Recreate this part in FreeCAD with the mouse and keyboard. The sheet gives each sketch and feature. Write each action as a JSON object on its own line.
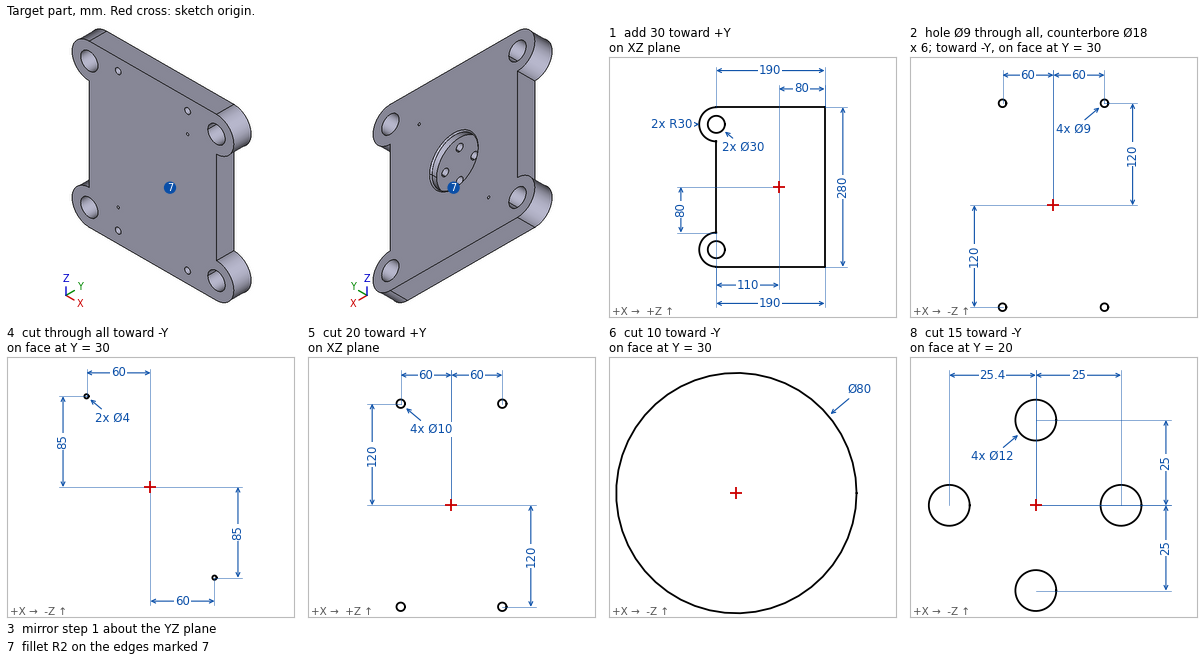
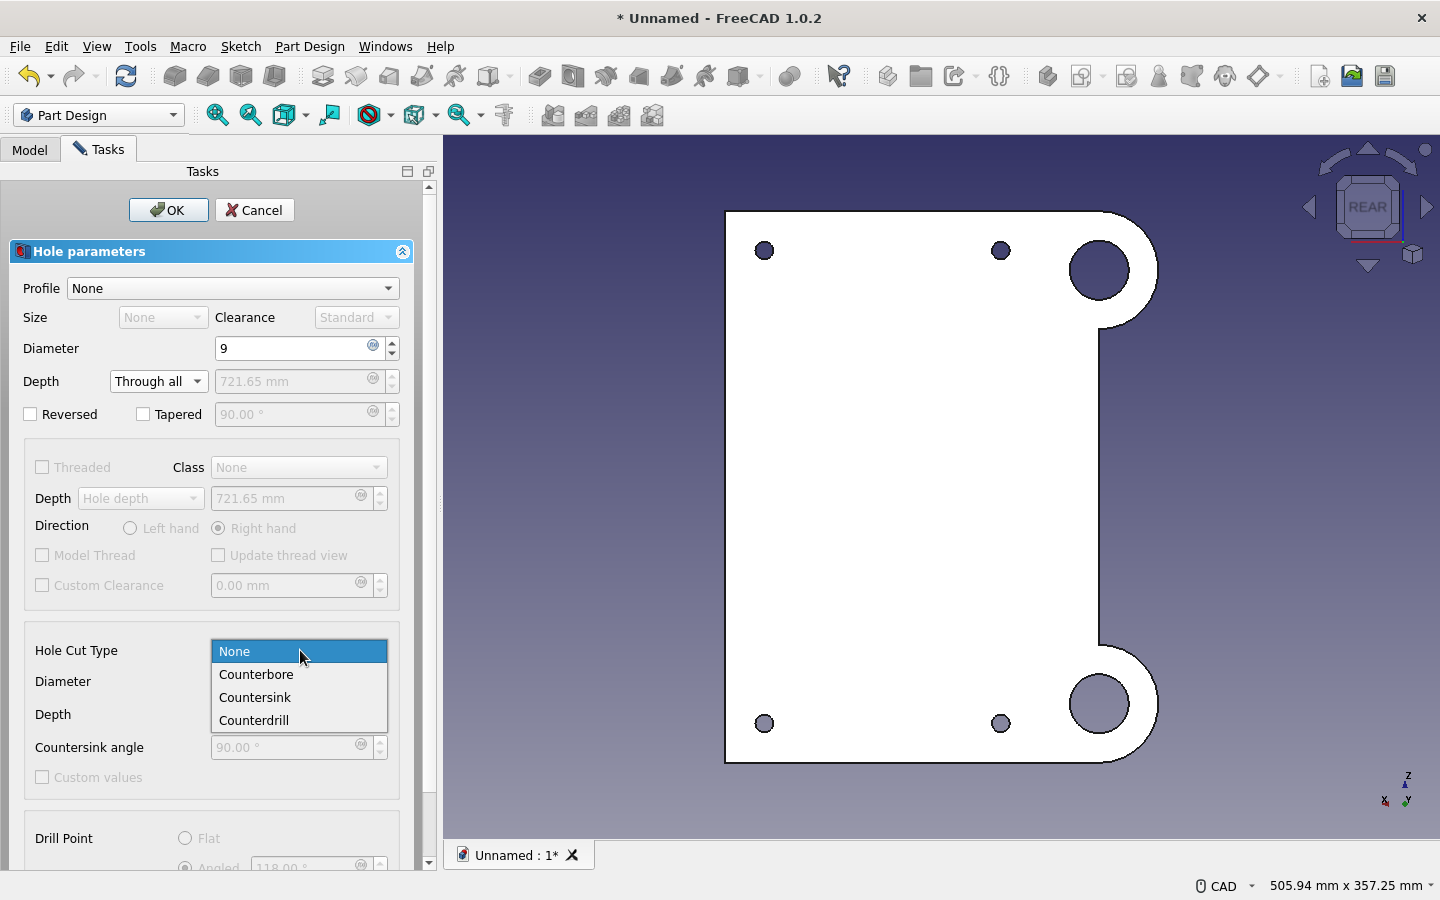
{"action": "left_click", "coordinate": [298, 674]}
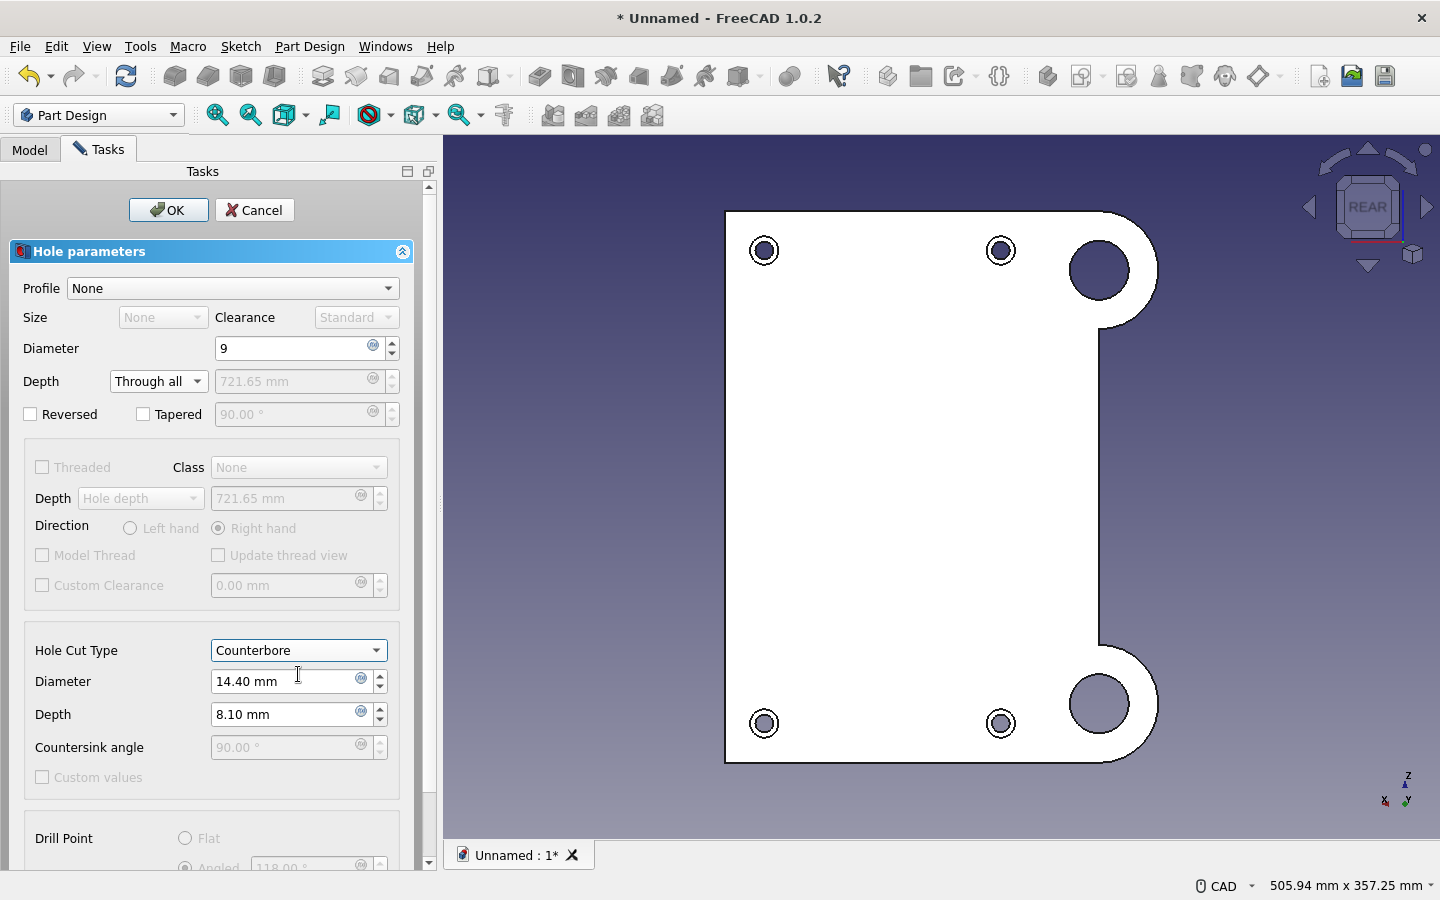
{"action": "triple_click", "coordinate": [292, 682]}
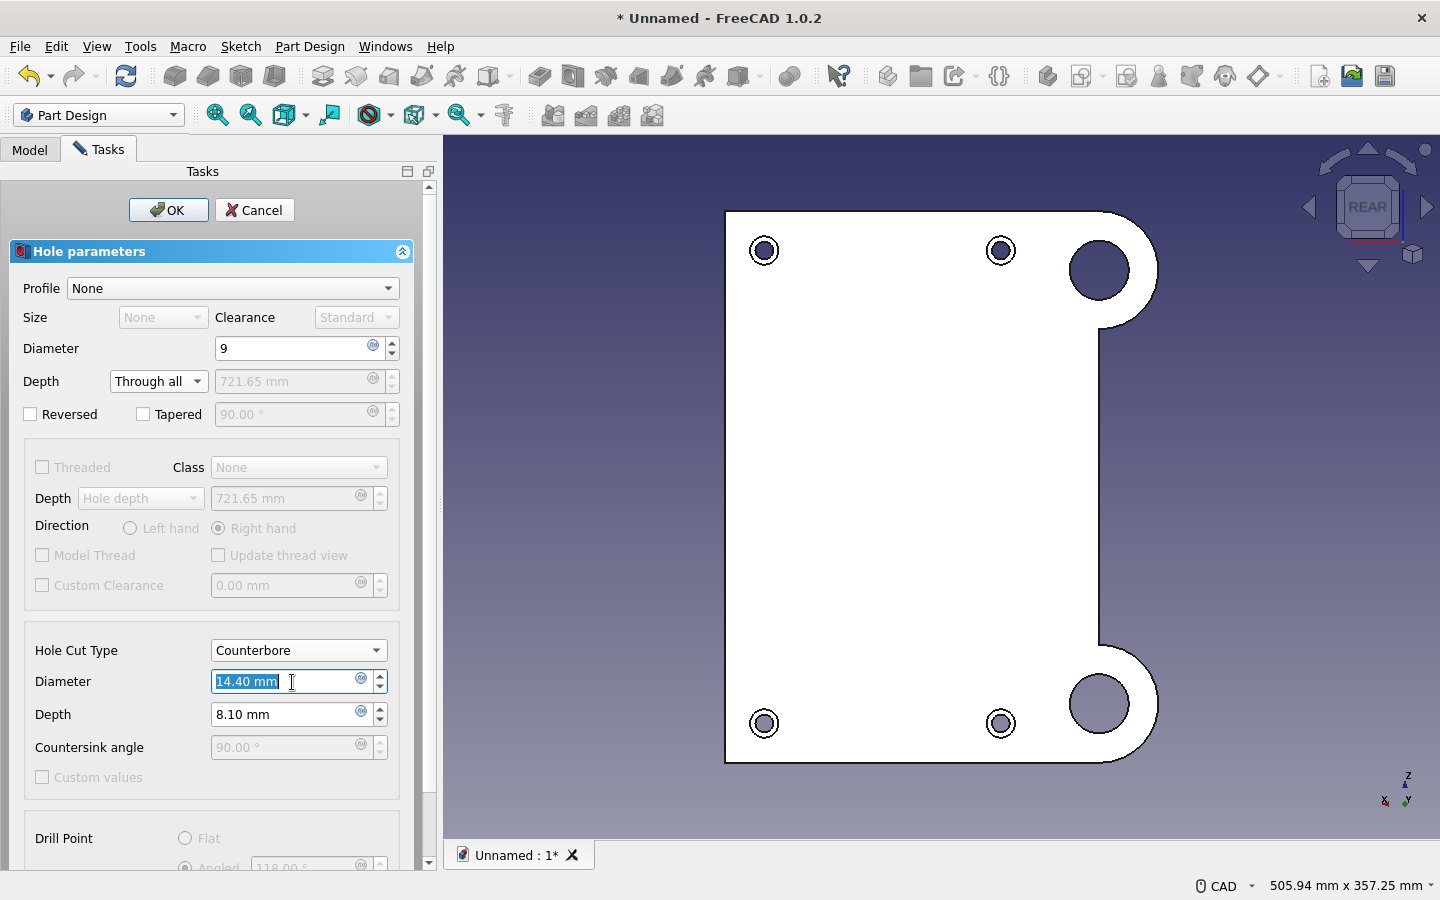
{"action": "type", "text": "18"}
{"action": "key", "text": "Tab"}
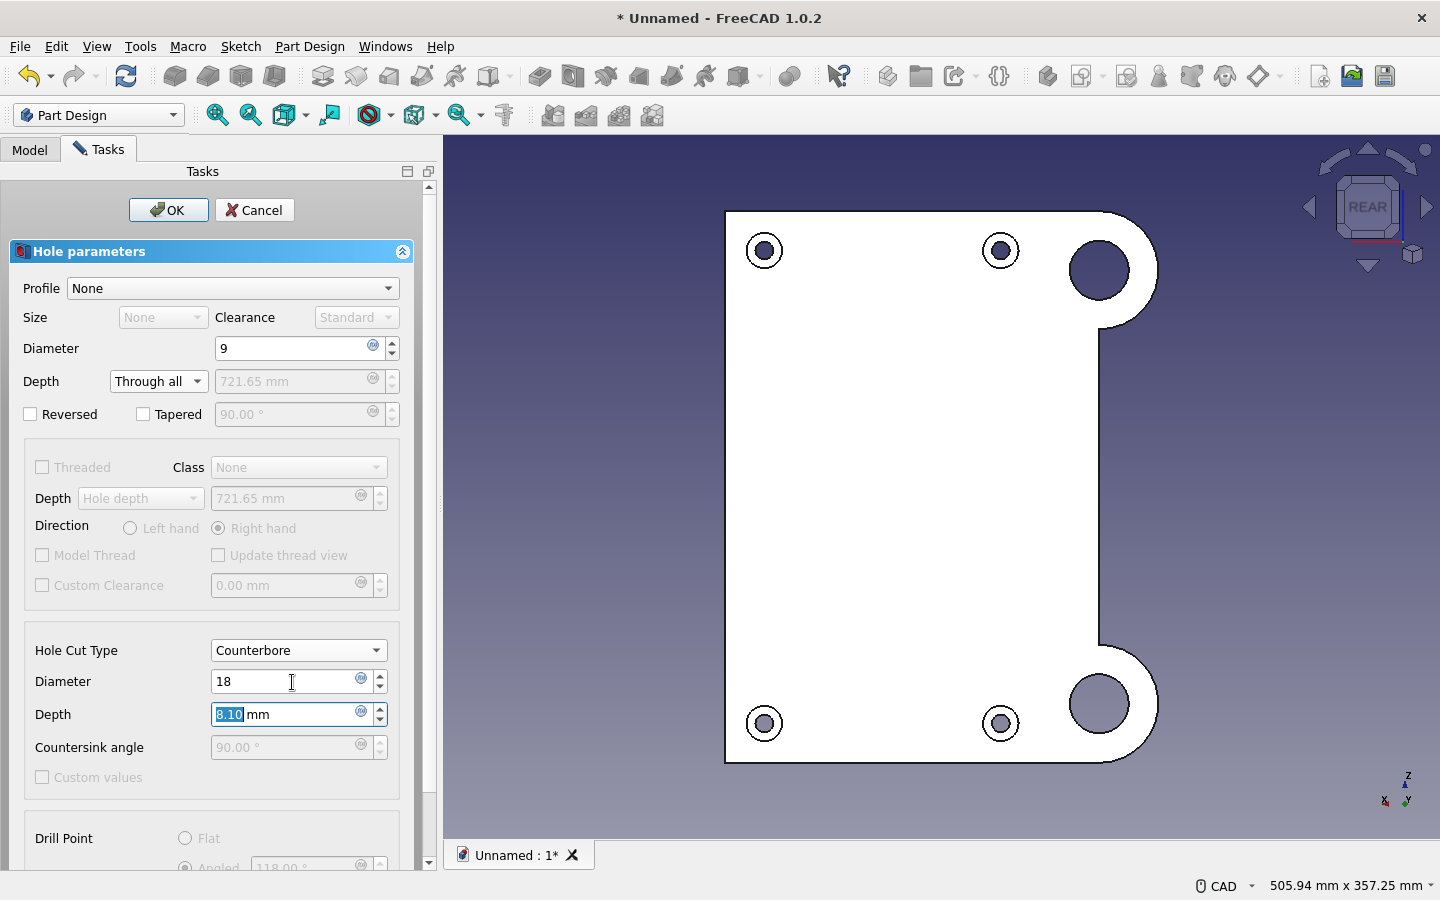
{"action": "type", "text": "6"}
{"action": "key", "text": "Tab"}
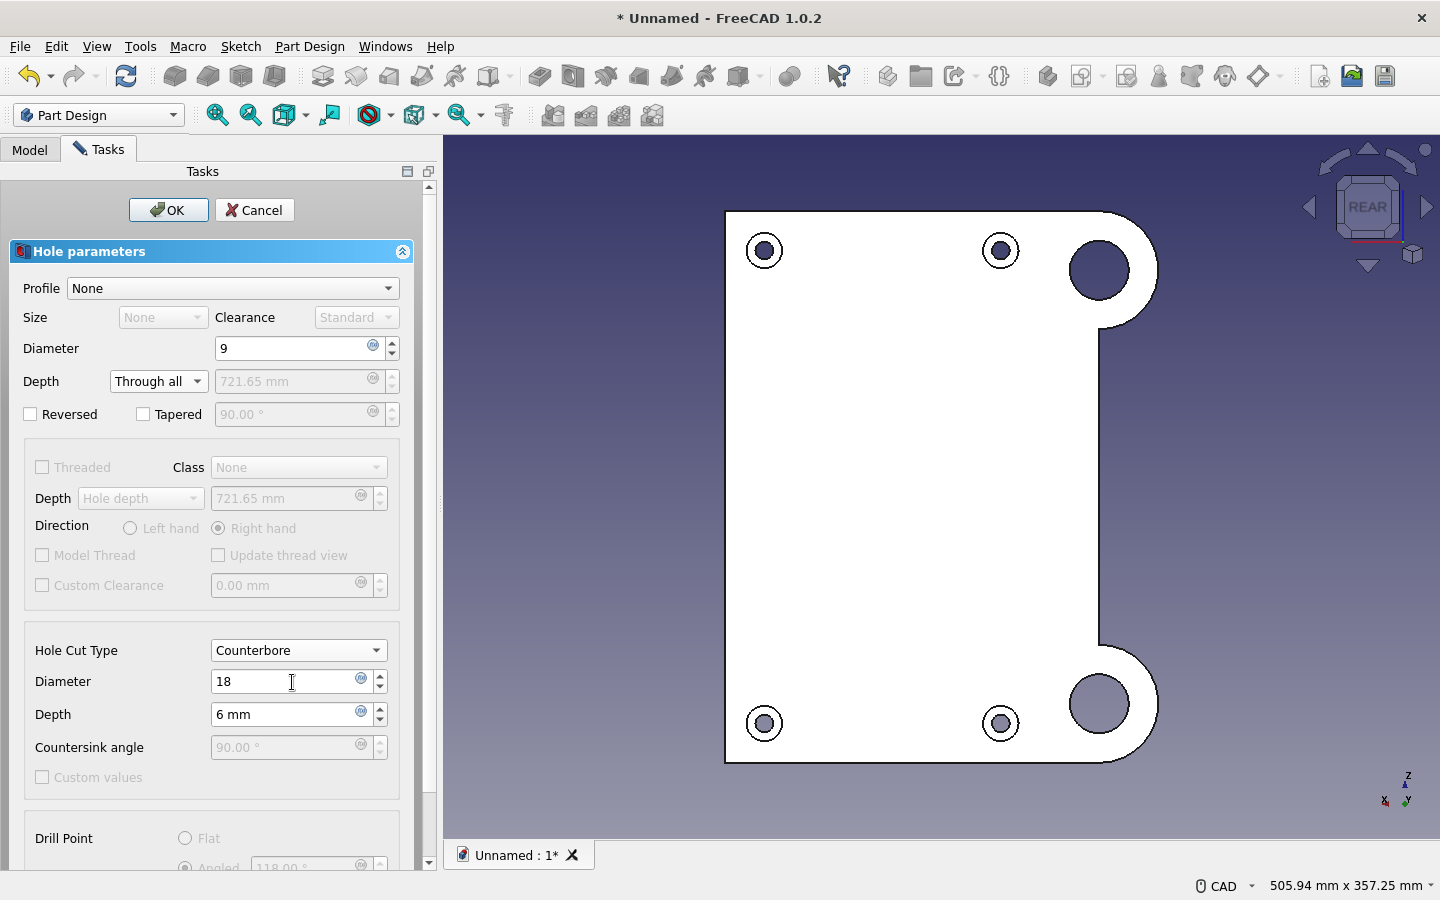
{"action": "left_click", "coordinate": [169, 210]}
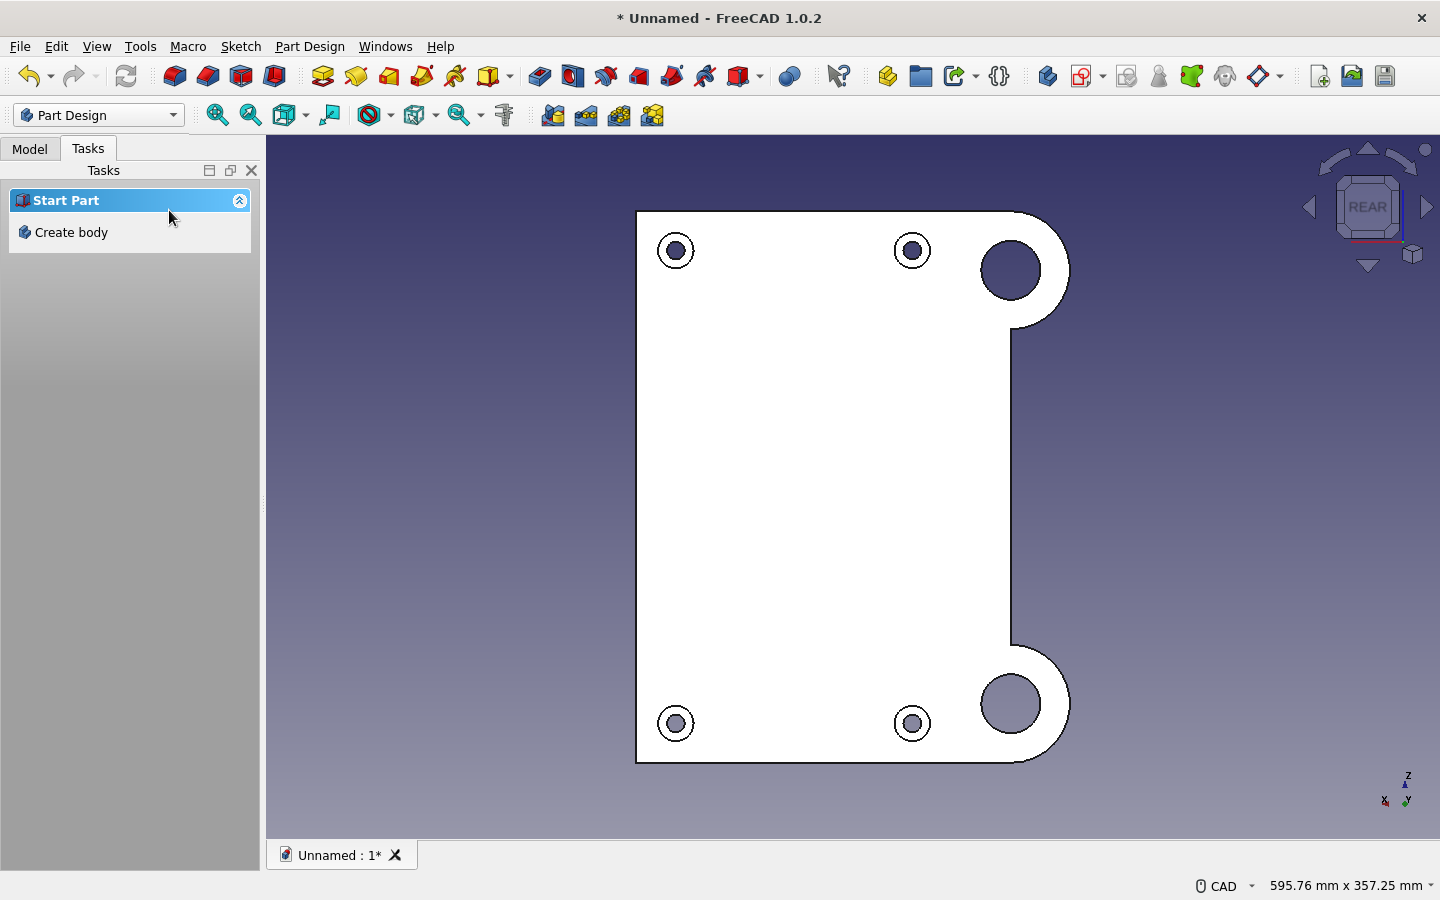
{"action": "left_click", "coordinate": [30, 148]}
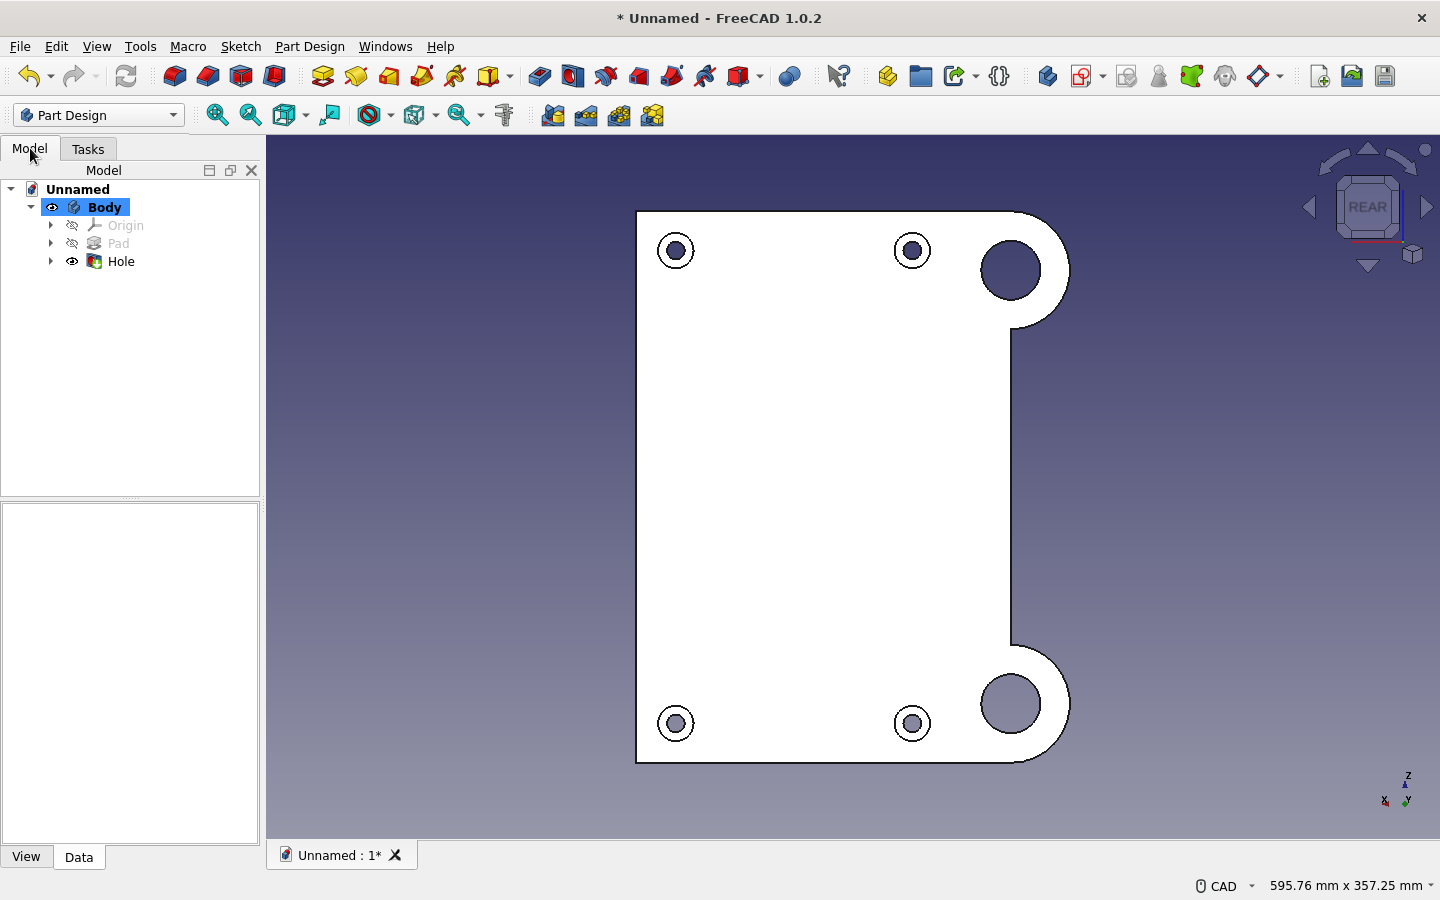
{"action": "left_click", "coordinate": [117, 243]}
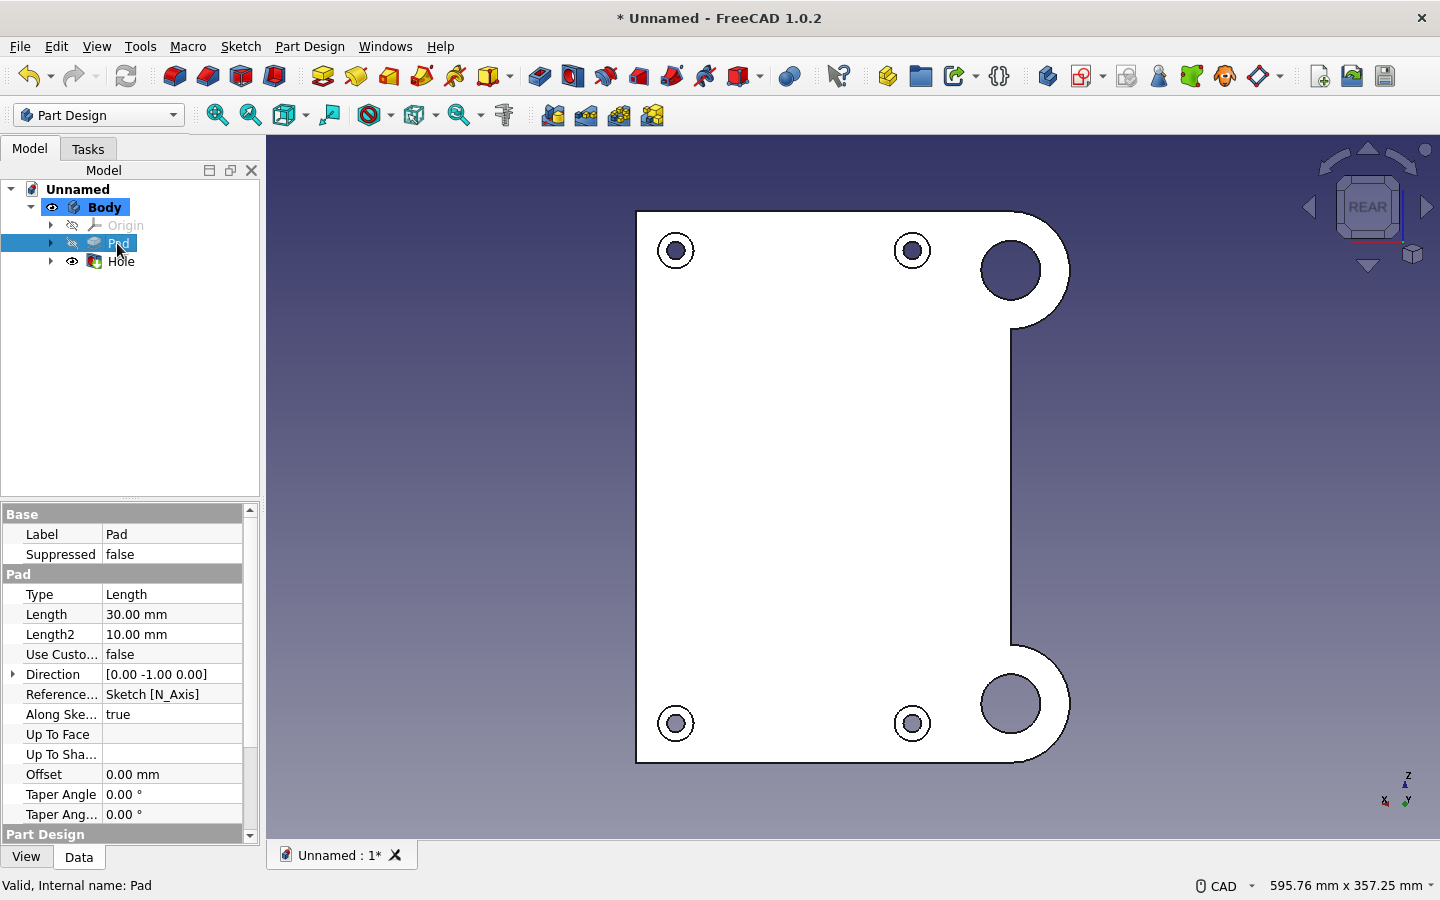
{"action": "left_click", "coordinate": [553, 116]}